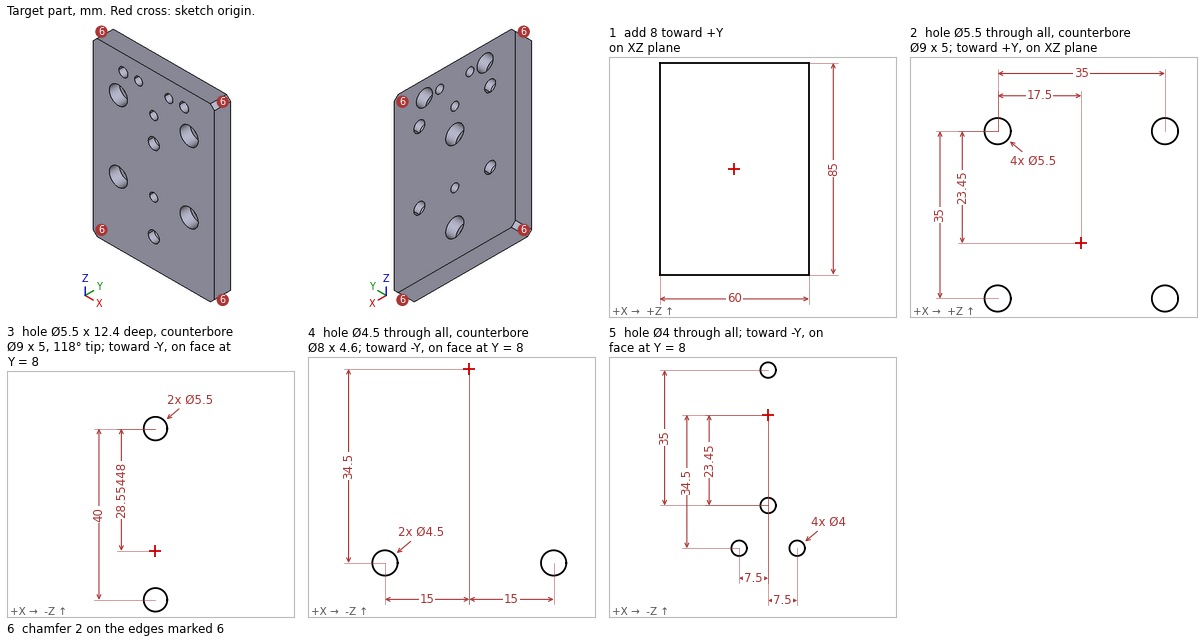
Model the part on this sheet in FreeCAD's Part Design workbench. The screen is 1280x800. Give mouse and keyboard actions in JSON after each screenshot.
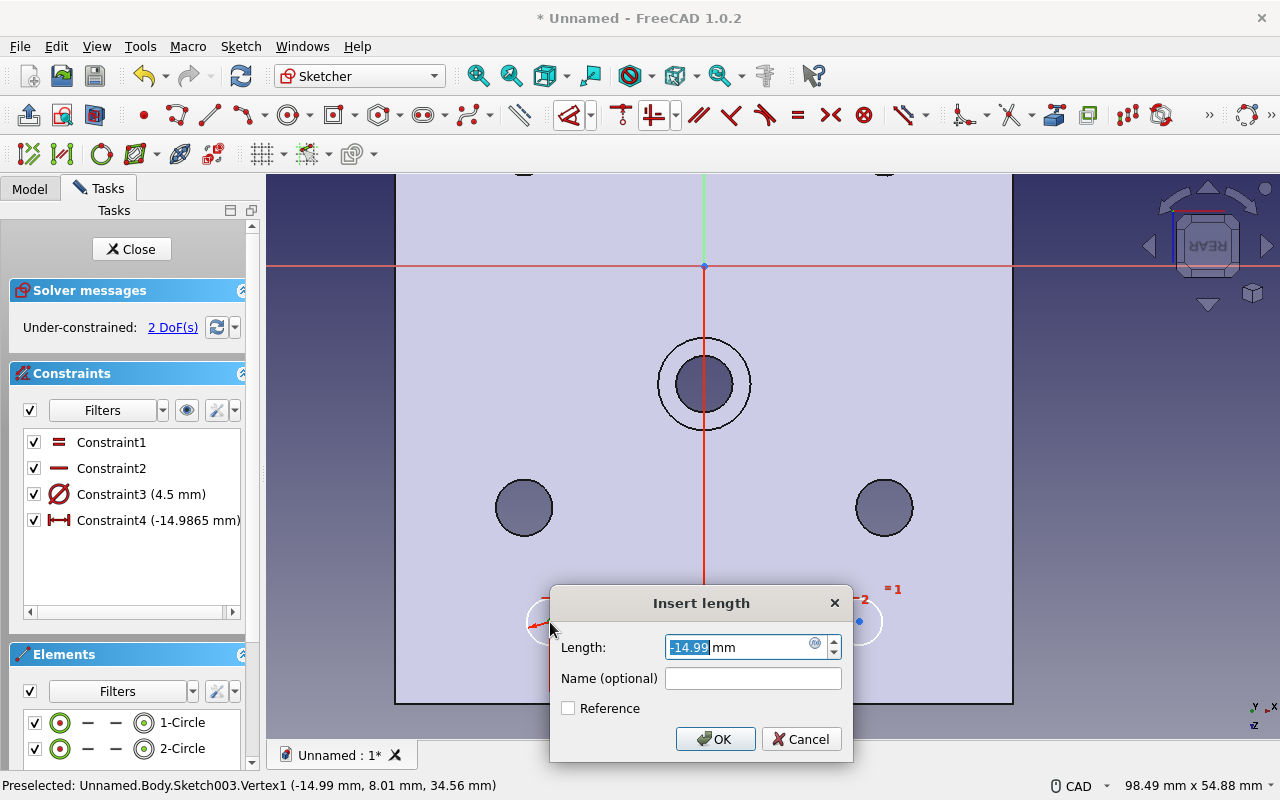
{"action": "type", "text": "-15"}
{"action": "key", "text": "Return"}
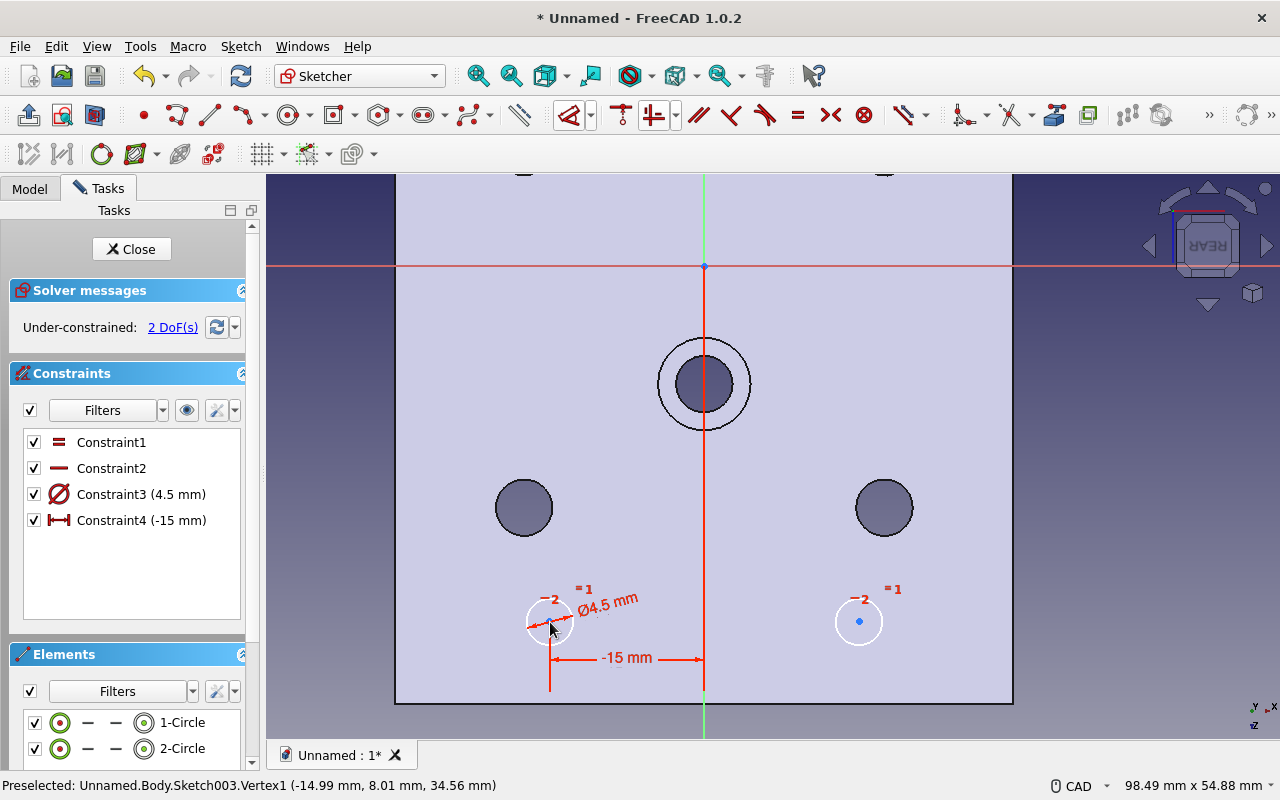
{"action": "left_click", "coordinate": [859, 622]}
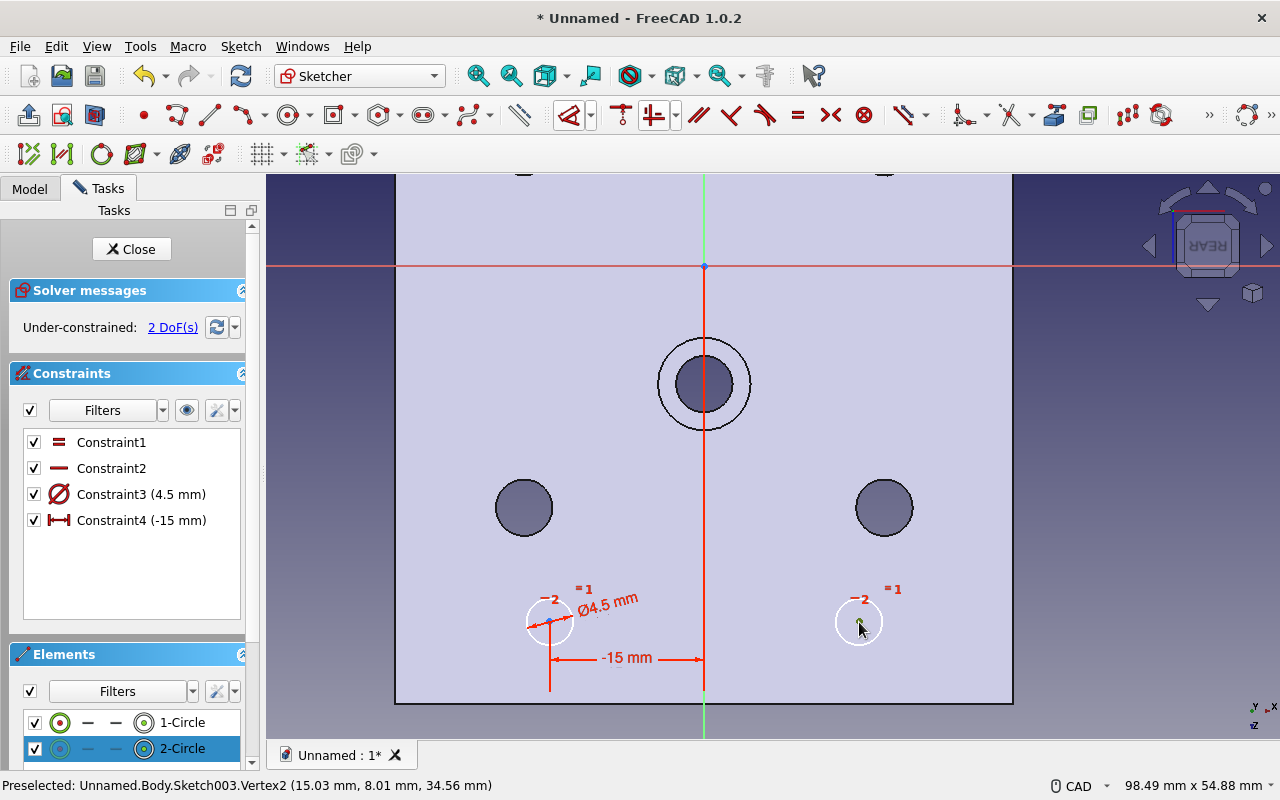
{"action": "key", "text": "l"}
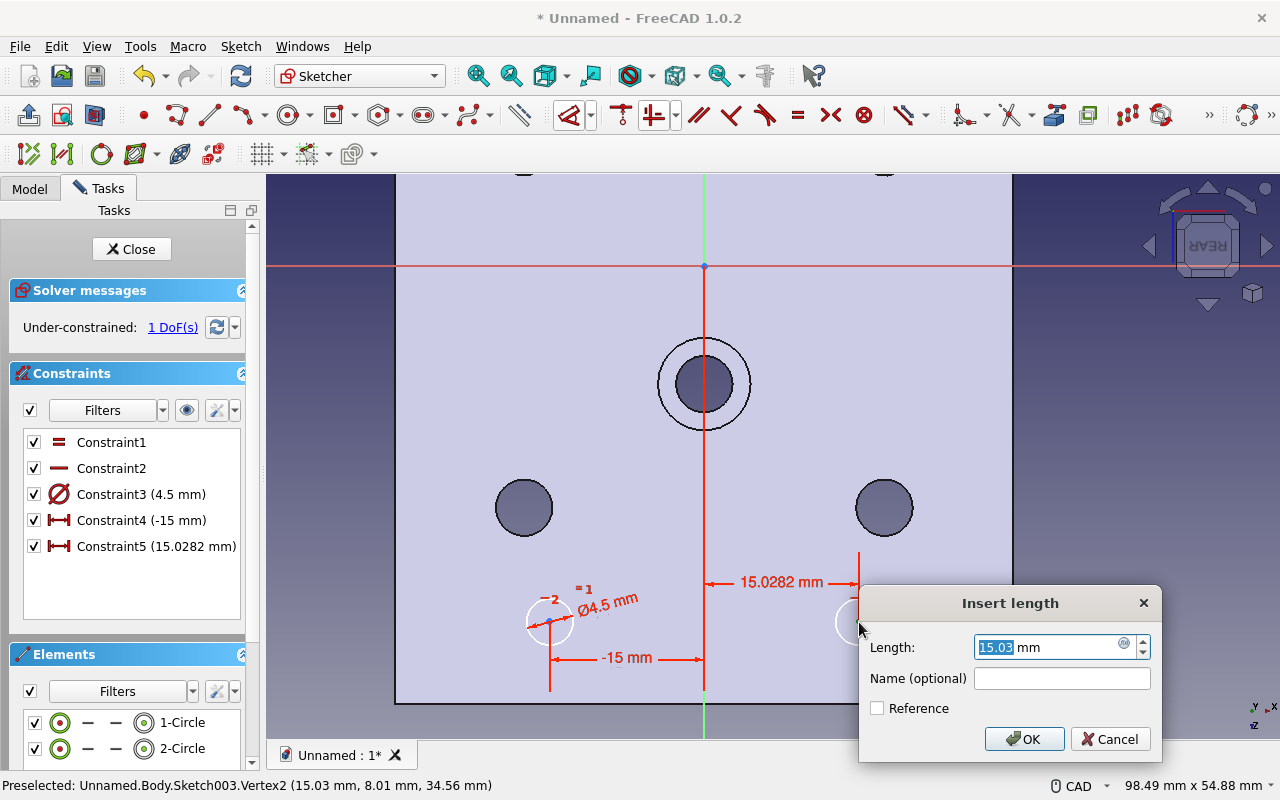
{"action": "type", "text": "15"}
{"action": "key", "text": "Return"}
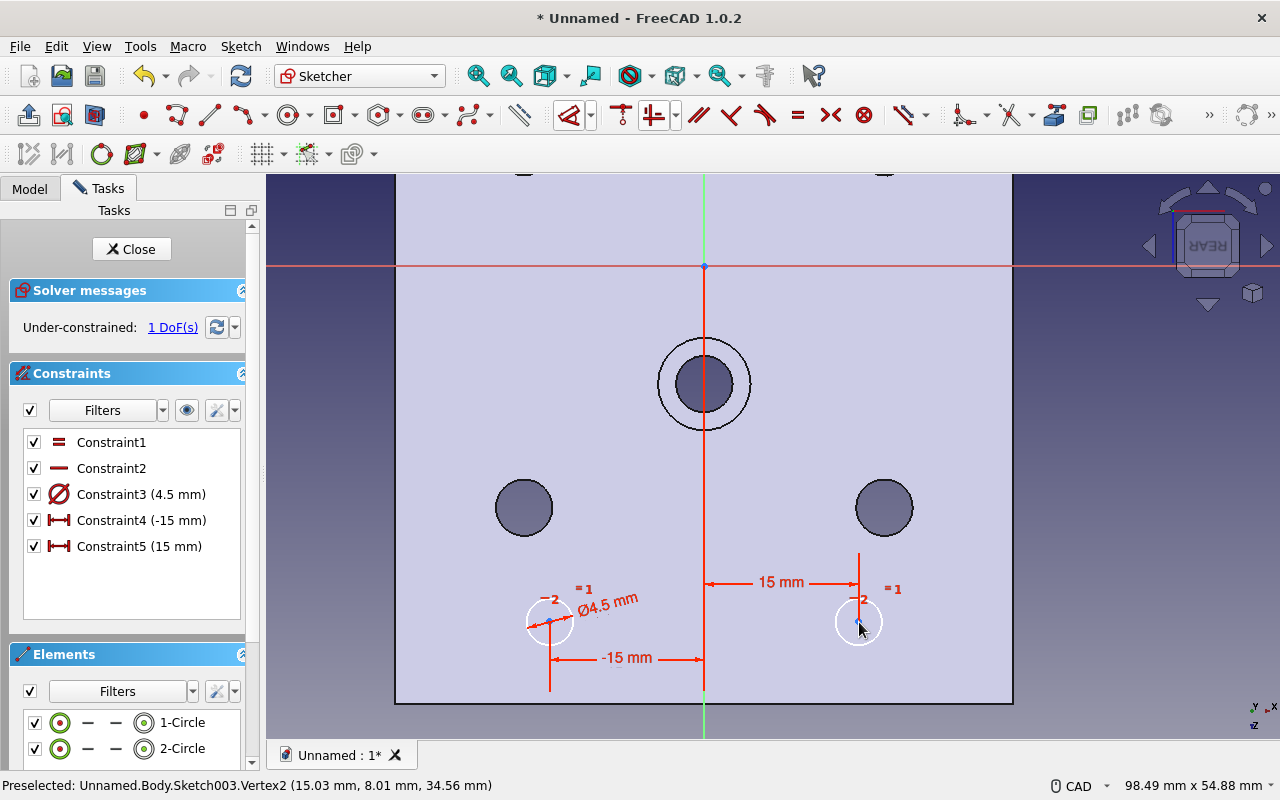
{"action": "left_click", "coordinate": [550, 622]}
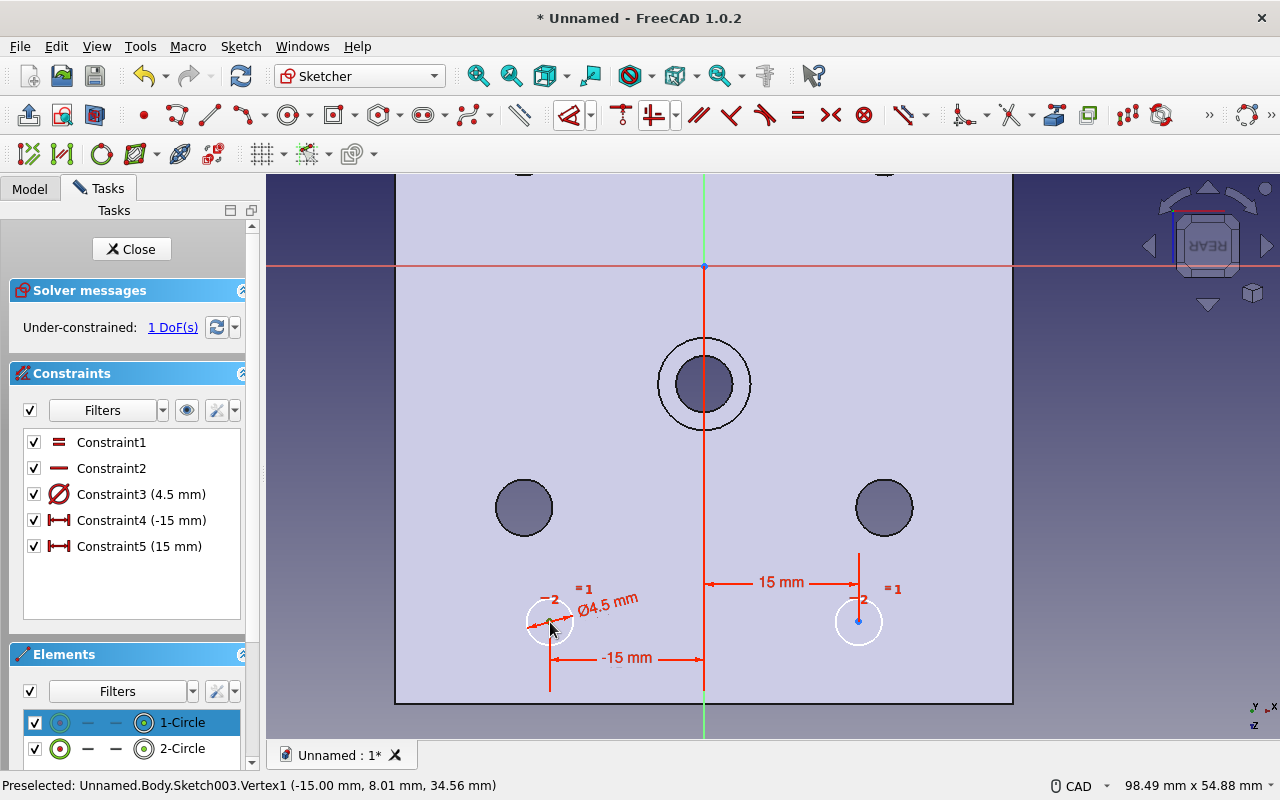
{"action": "left_click", "coordinate": [590, 116]}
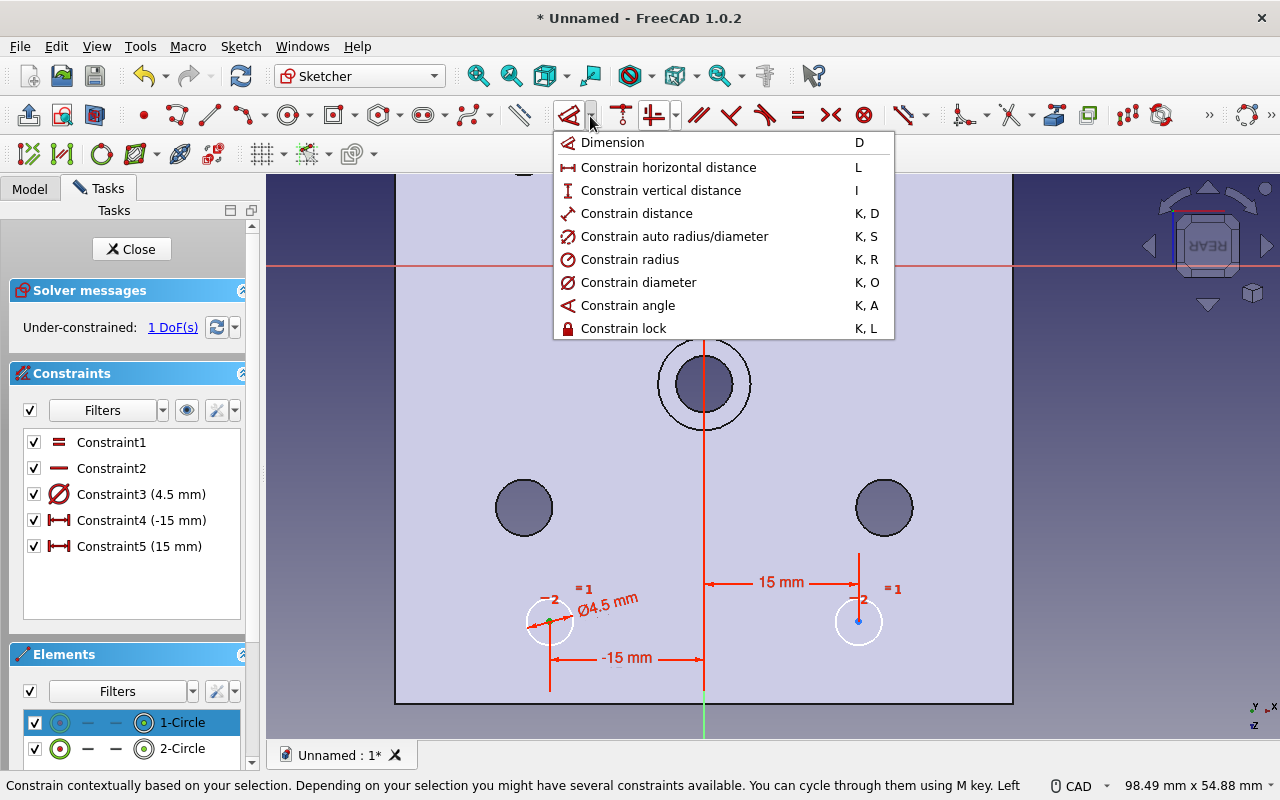
{"action": "left_click", "coordinate": [724, 190]}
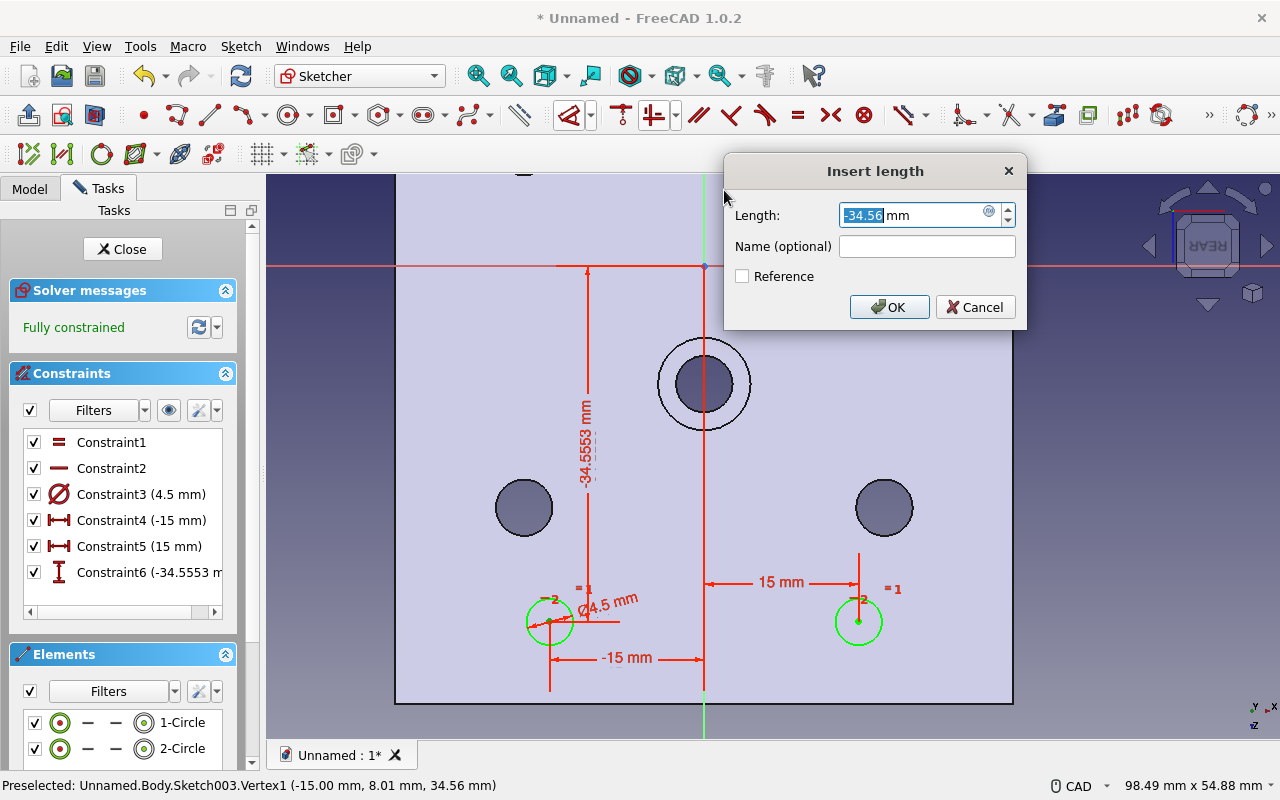
{"action": "type", "text": "-34.5"}
{"action": "key", "text": "Return"}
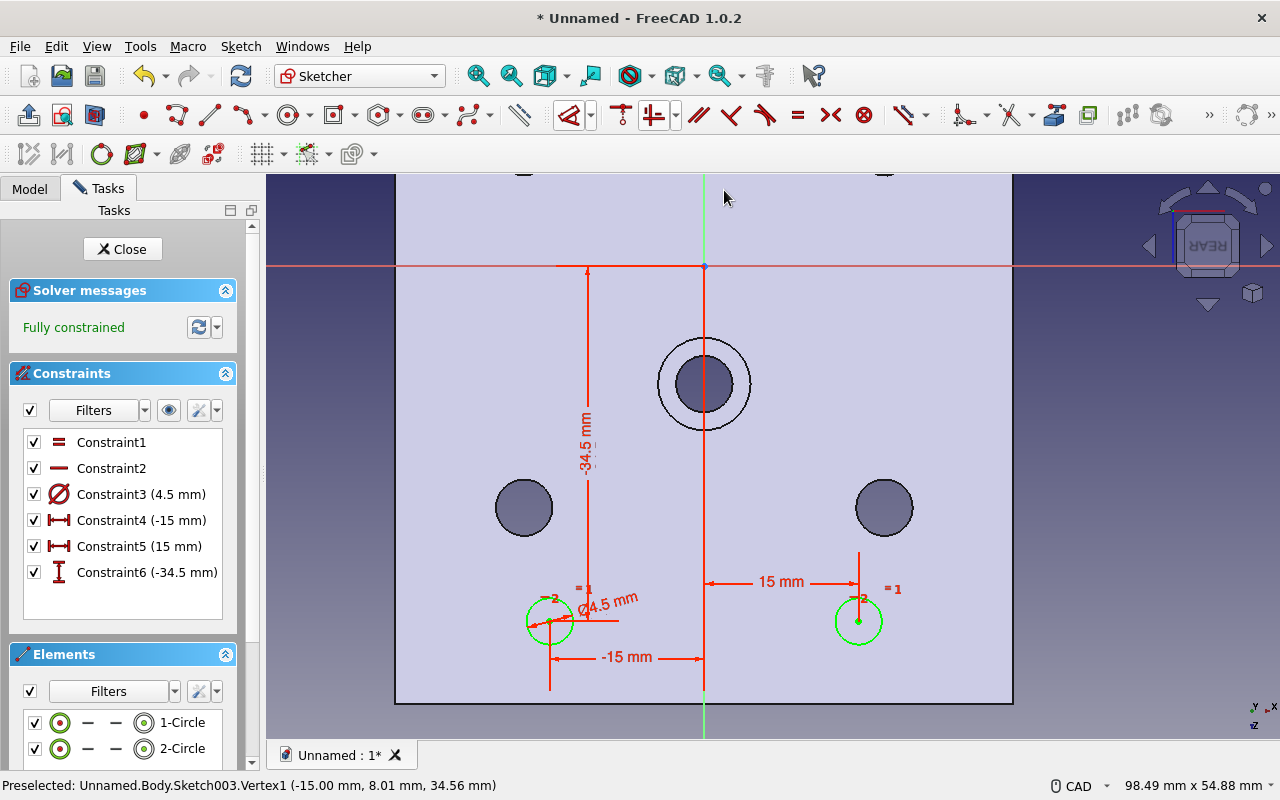
{"action": "left_click", "coordinate": [123, 249]}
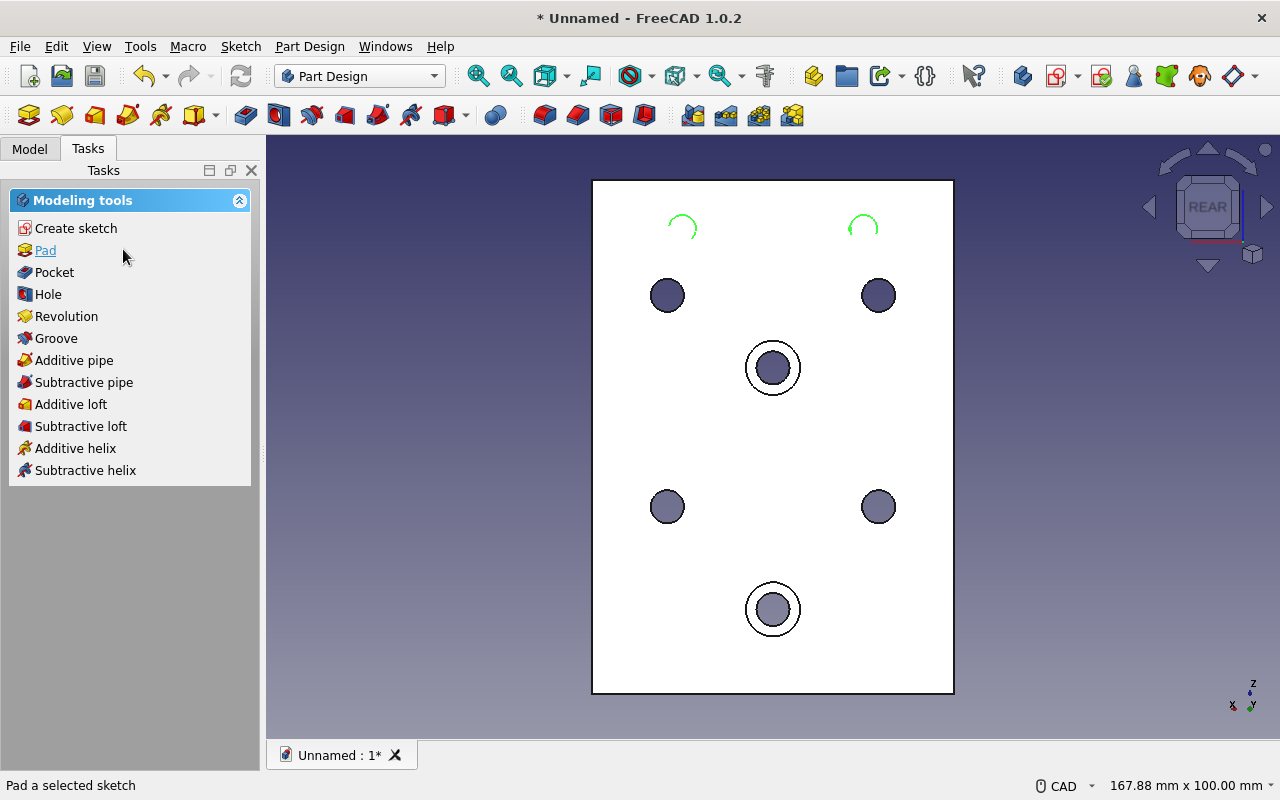
{"action": "left_click", "coordinate": [279, 116]}